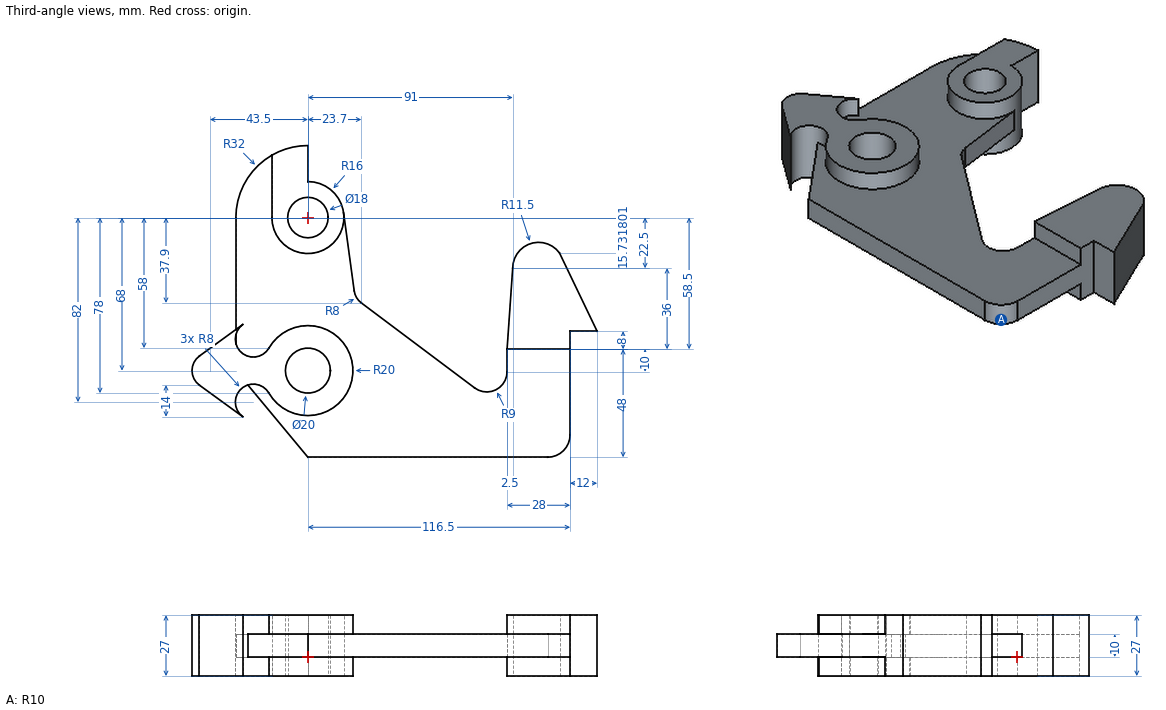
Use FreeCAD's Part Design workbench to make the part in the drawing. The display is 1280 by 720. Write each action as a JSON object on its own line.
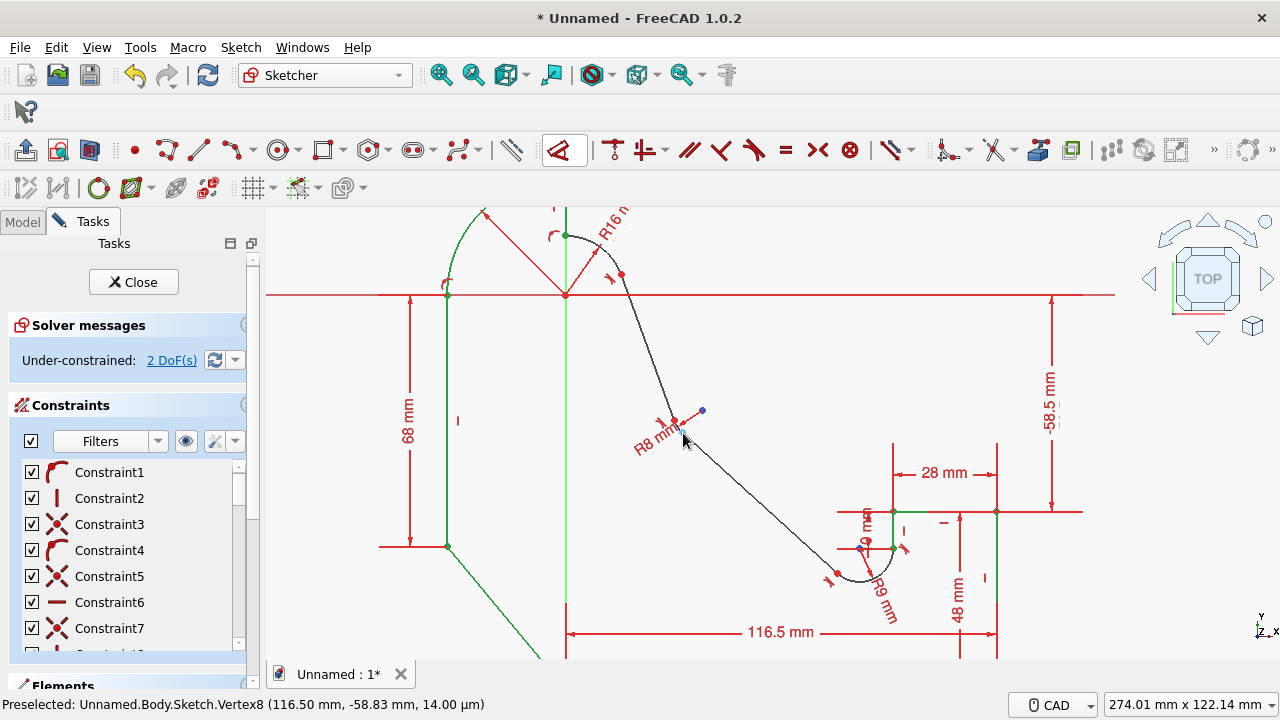
{"action": "left_click", "coordinate": [682, 432]}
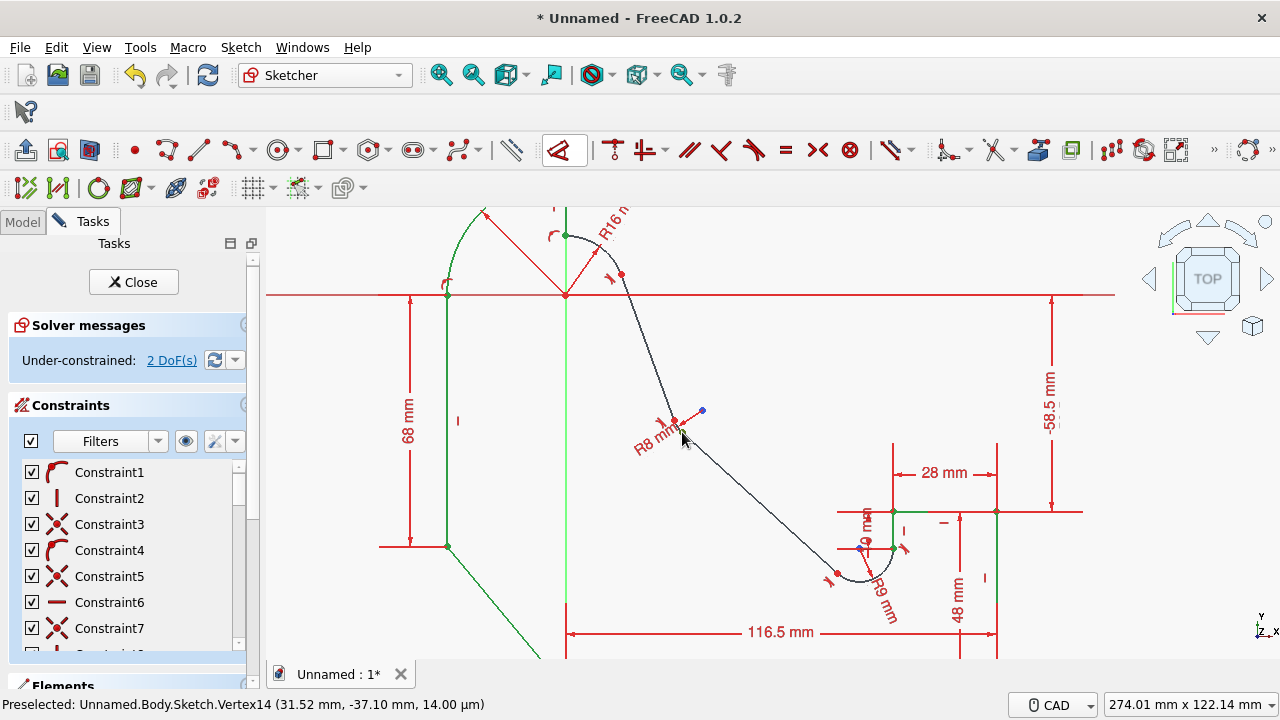
{"action": "left_click", "coordinate": [582, 150]}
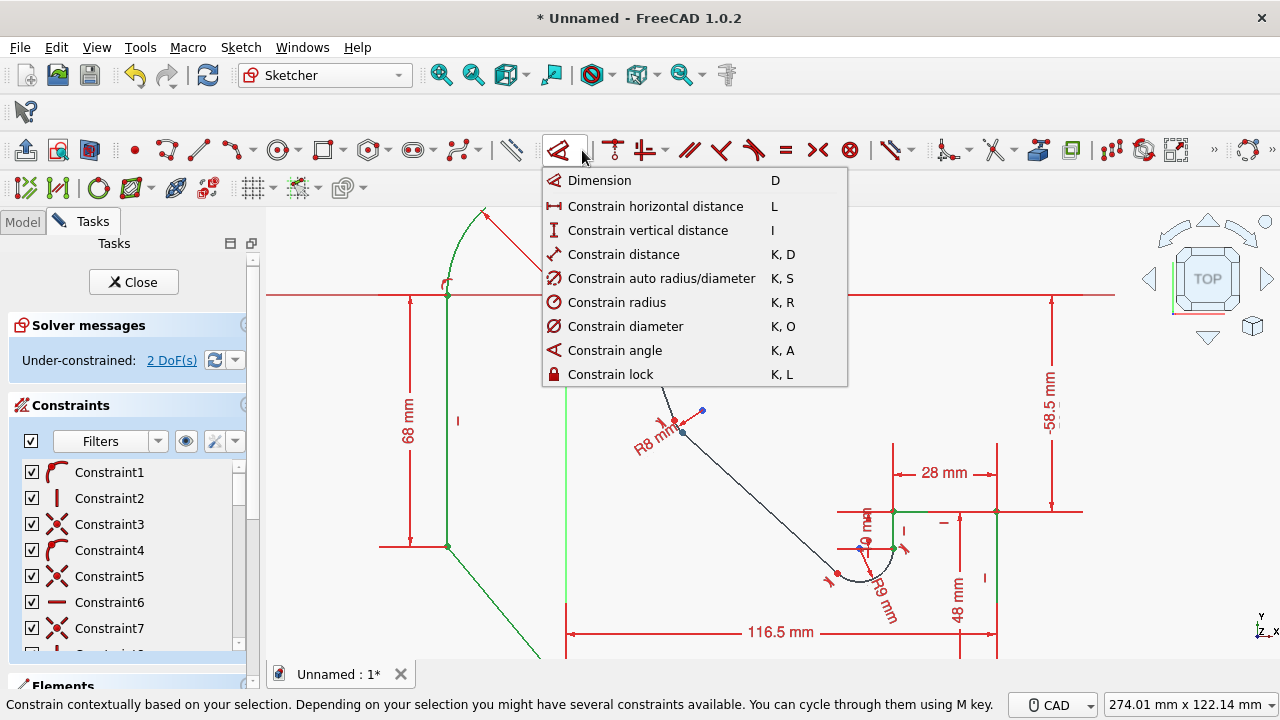
{"action": "left_click", "coordinate": [695, 206]}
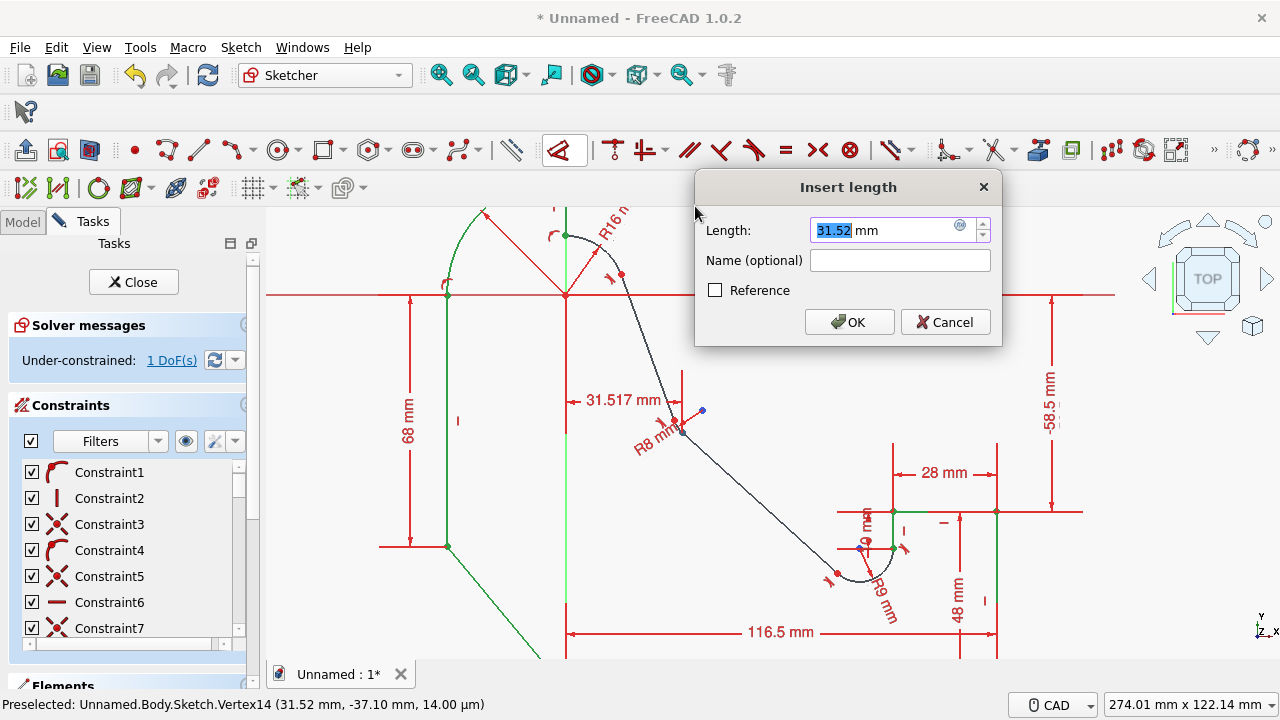
{"action": "type", "text": "23.7"}
{"action": "key", "text": "Return"}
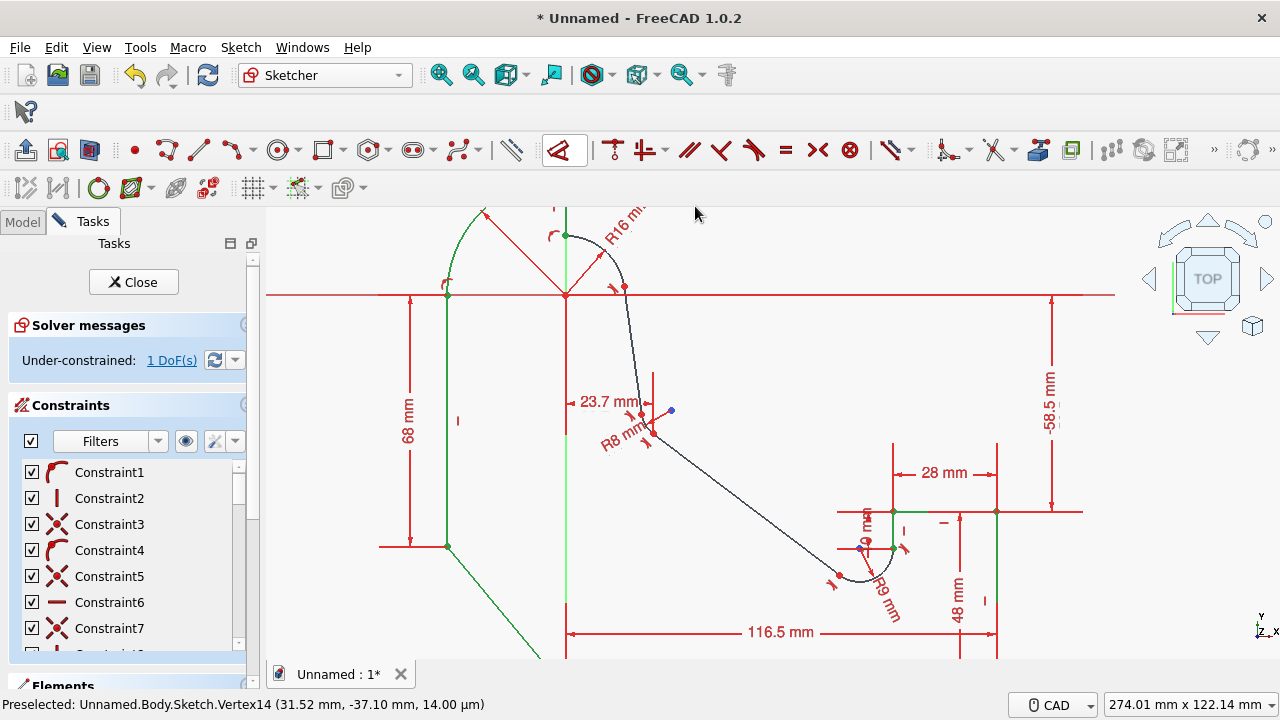
{"action": "left_click", "coordinate": [653, 434]}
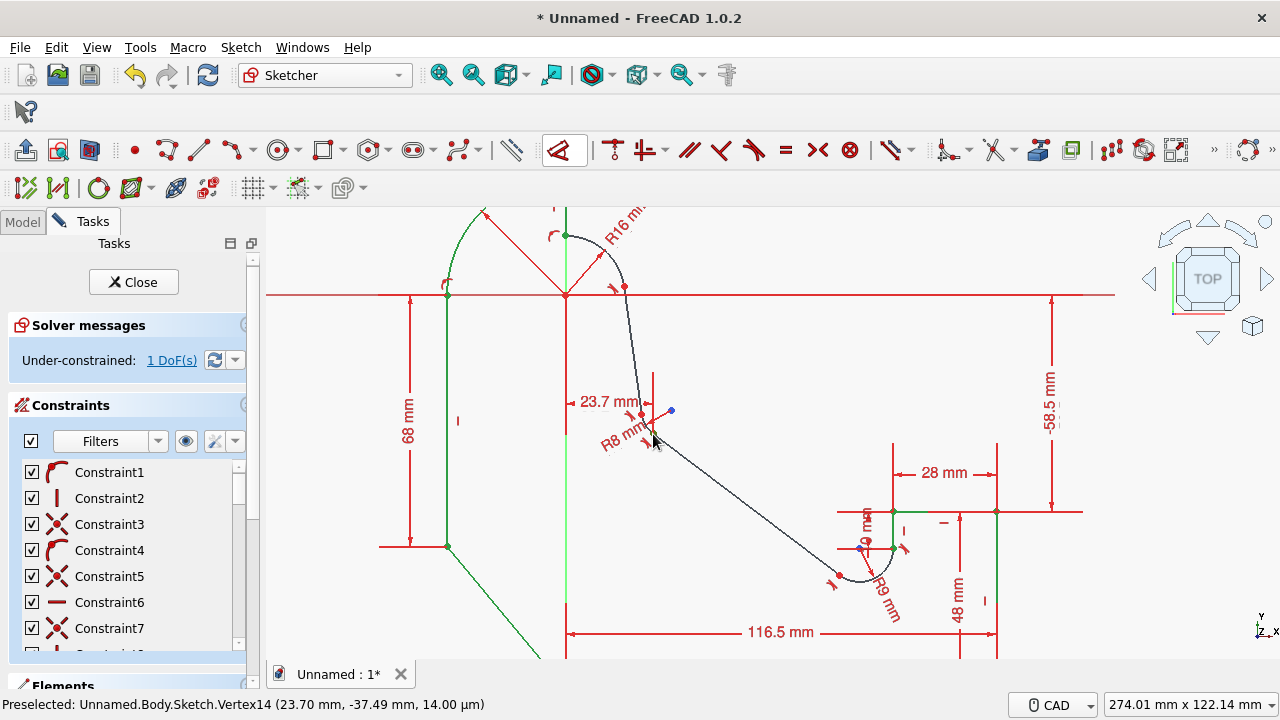
{"action": "key", "text": "i"}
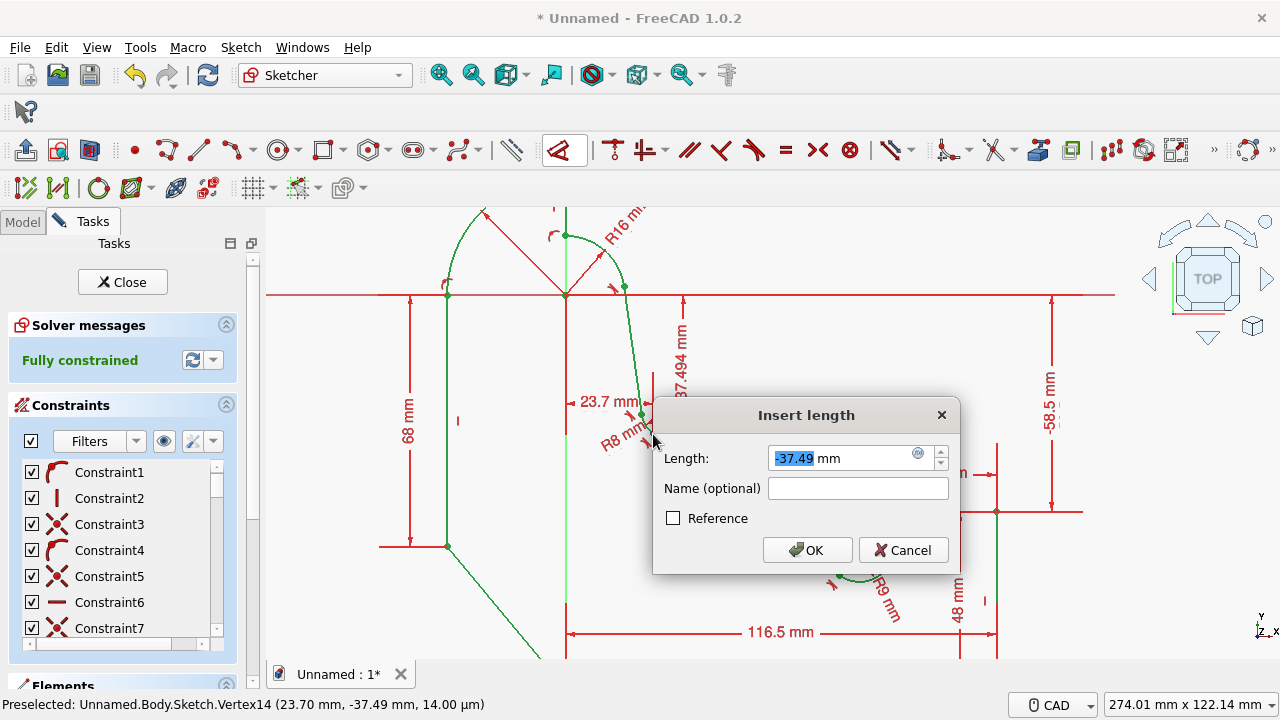
{"action": "type", "text": "-37.9"}
{"action": "key", "text": "Return"}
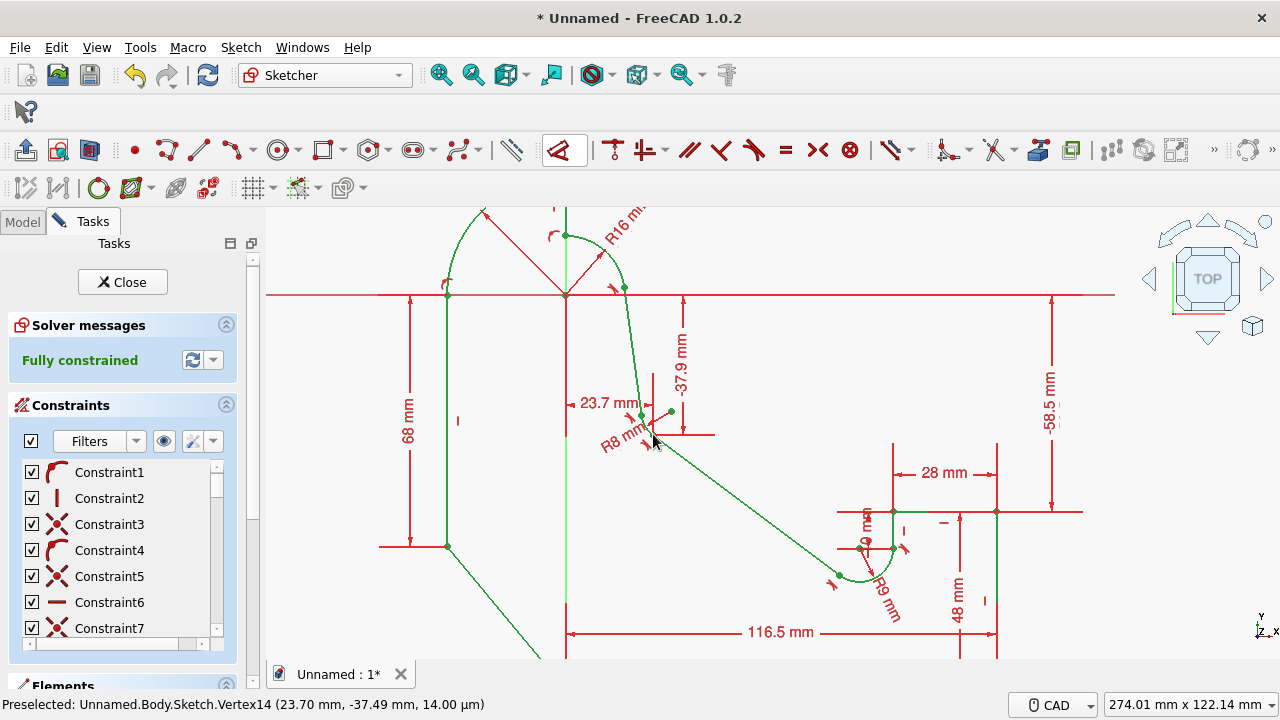
{"action": "left_click", "coordinate": [123, 282]}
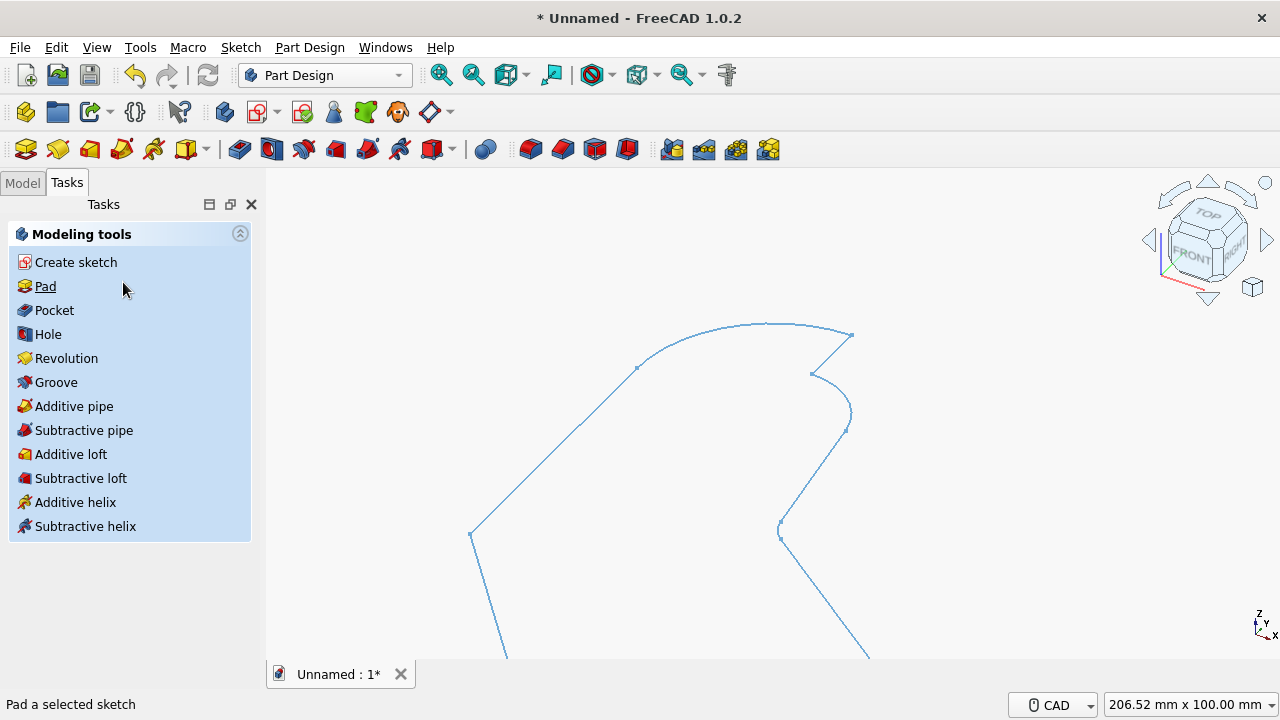
{"action": "left_click", "coordinate": [26, 150]}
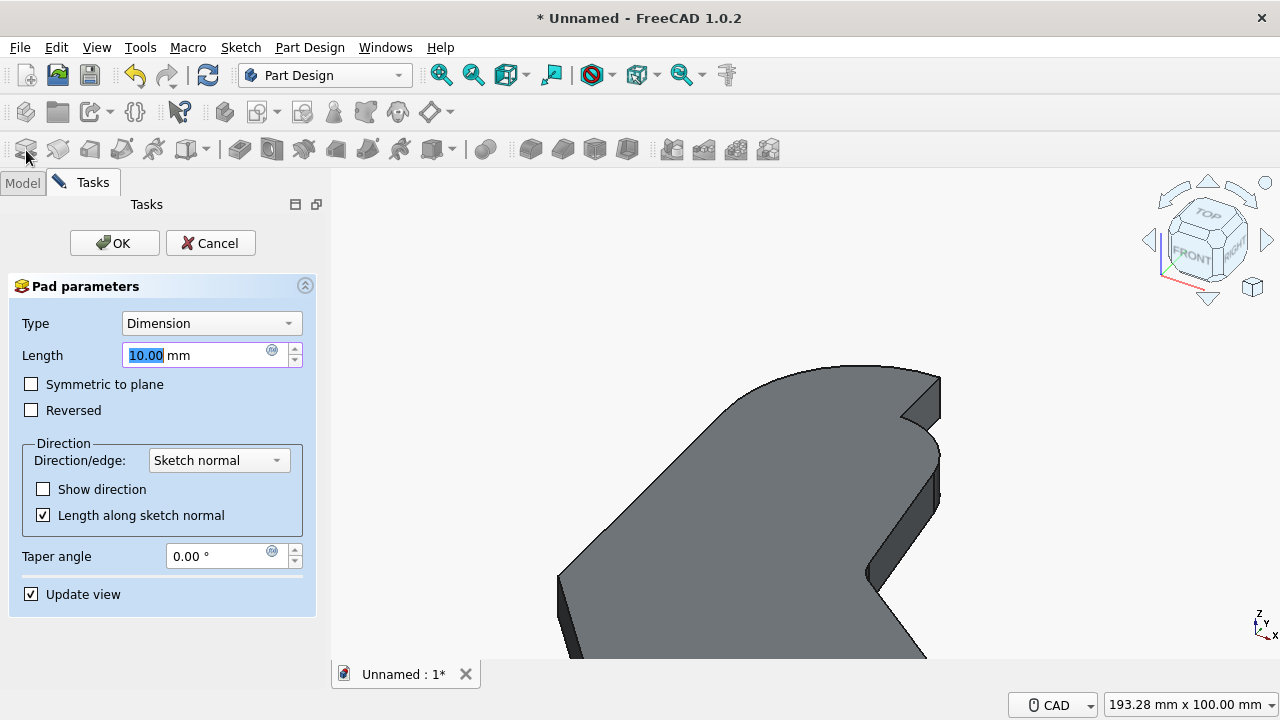
{"action": "type", "text": "10"}
{"action": "key", "text": "Tab"}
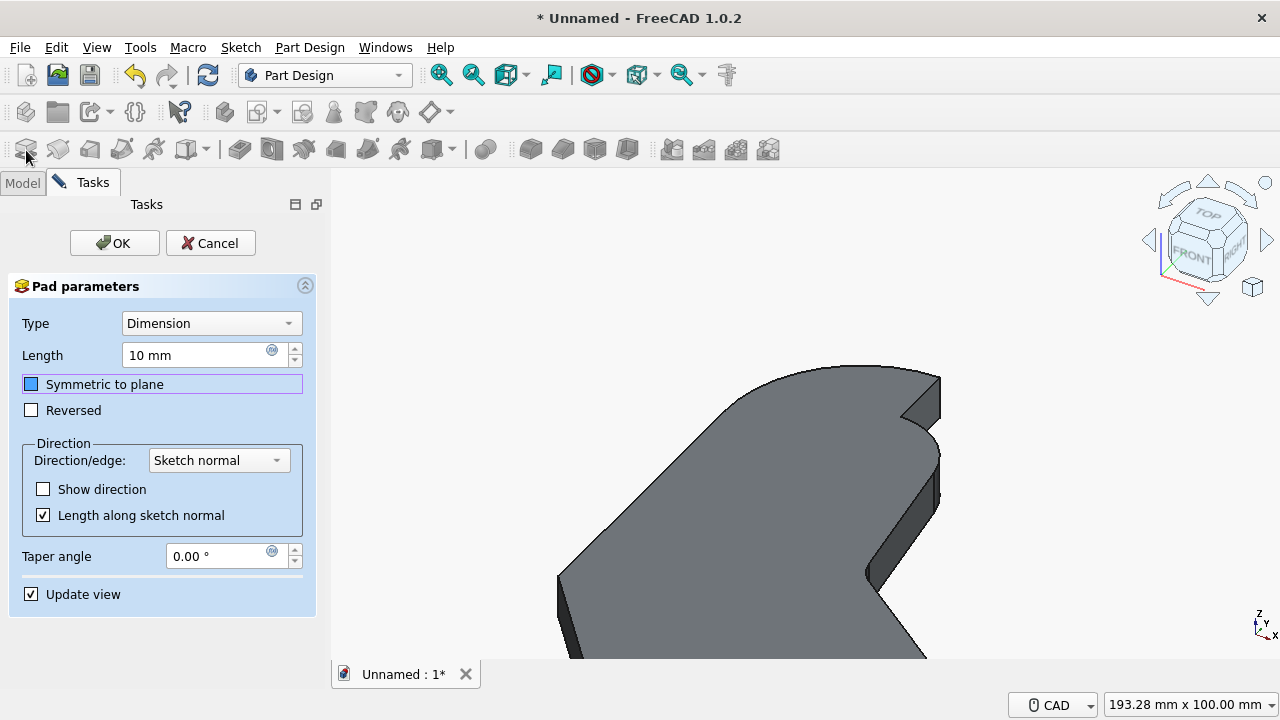
{"action": "left_click", "coordinate": [115, 243]}